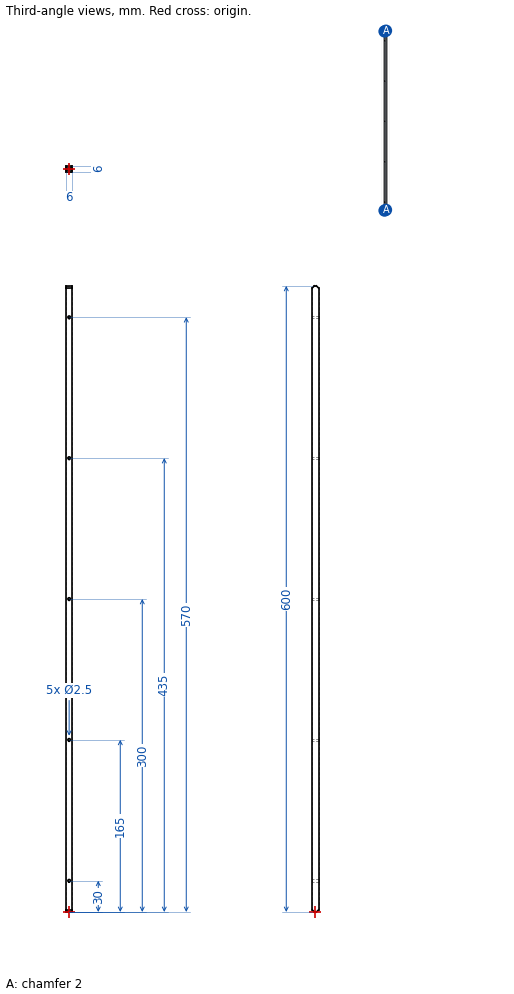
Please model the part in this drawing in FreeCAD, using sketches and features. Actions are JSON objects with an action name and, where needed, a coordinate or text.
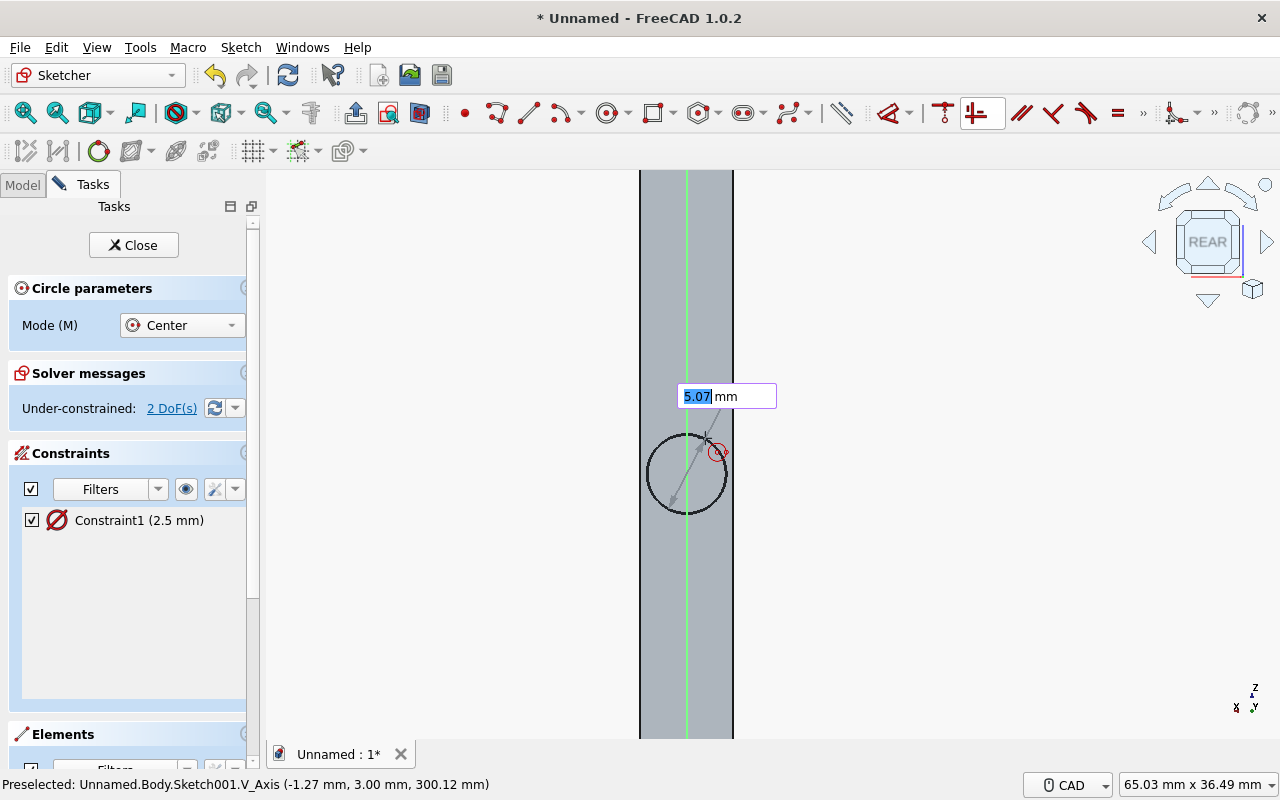
{"action": "type", "text": "2.5"}
{"action": "key", "text": "Return"}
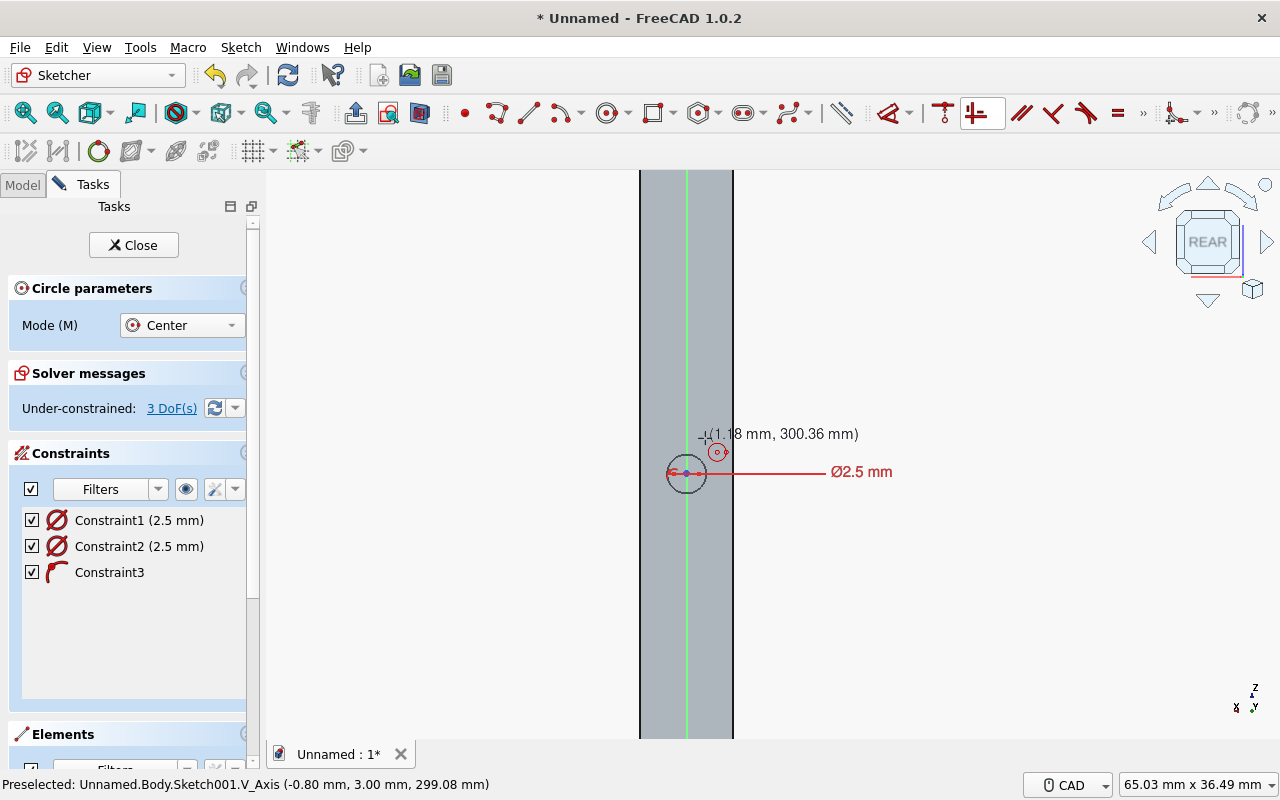
{"action": "scroll", "coordinate": [705, 443], "scroll_direction": "down", "scroll_amount": 15}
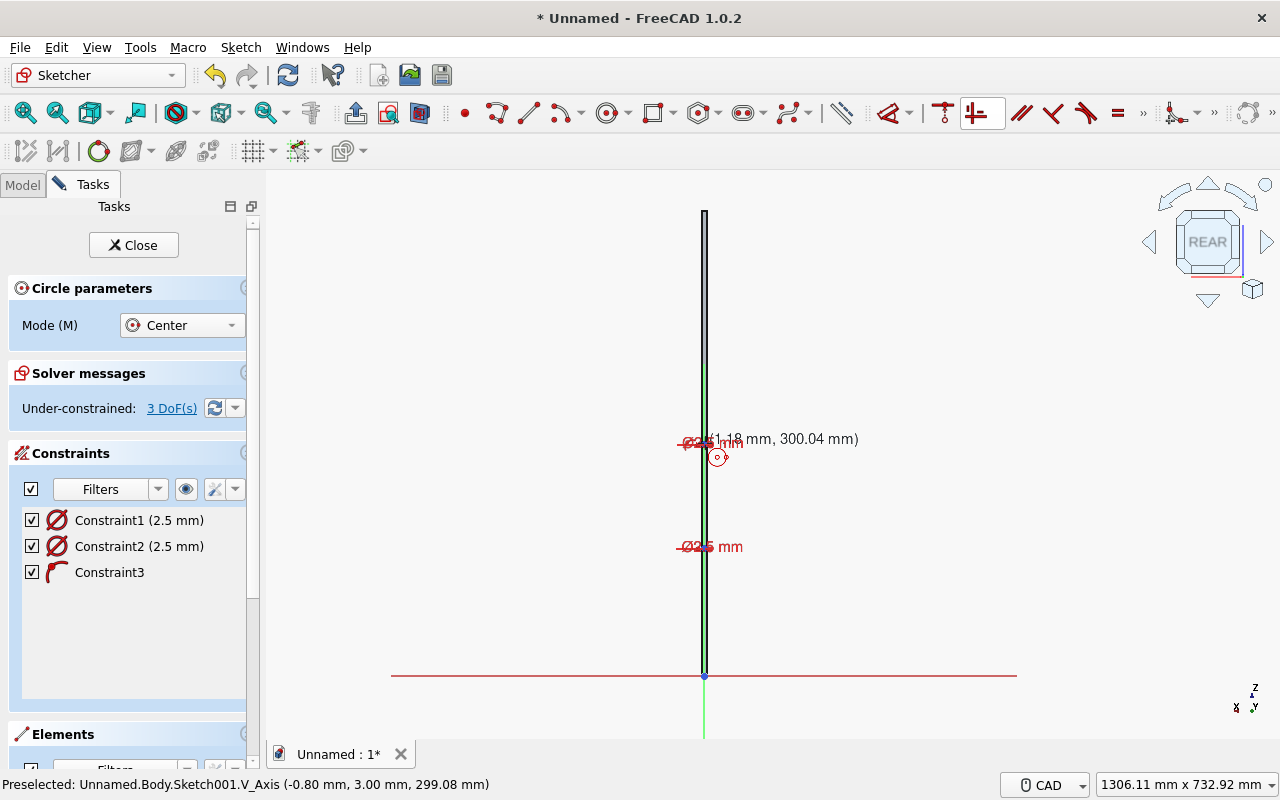
{"action": "scroll", "coordinate": [704, 339], "scroll_direction": "up", "scroll_amount": 16}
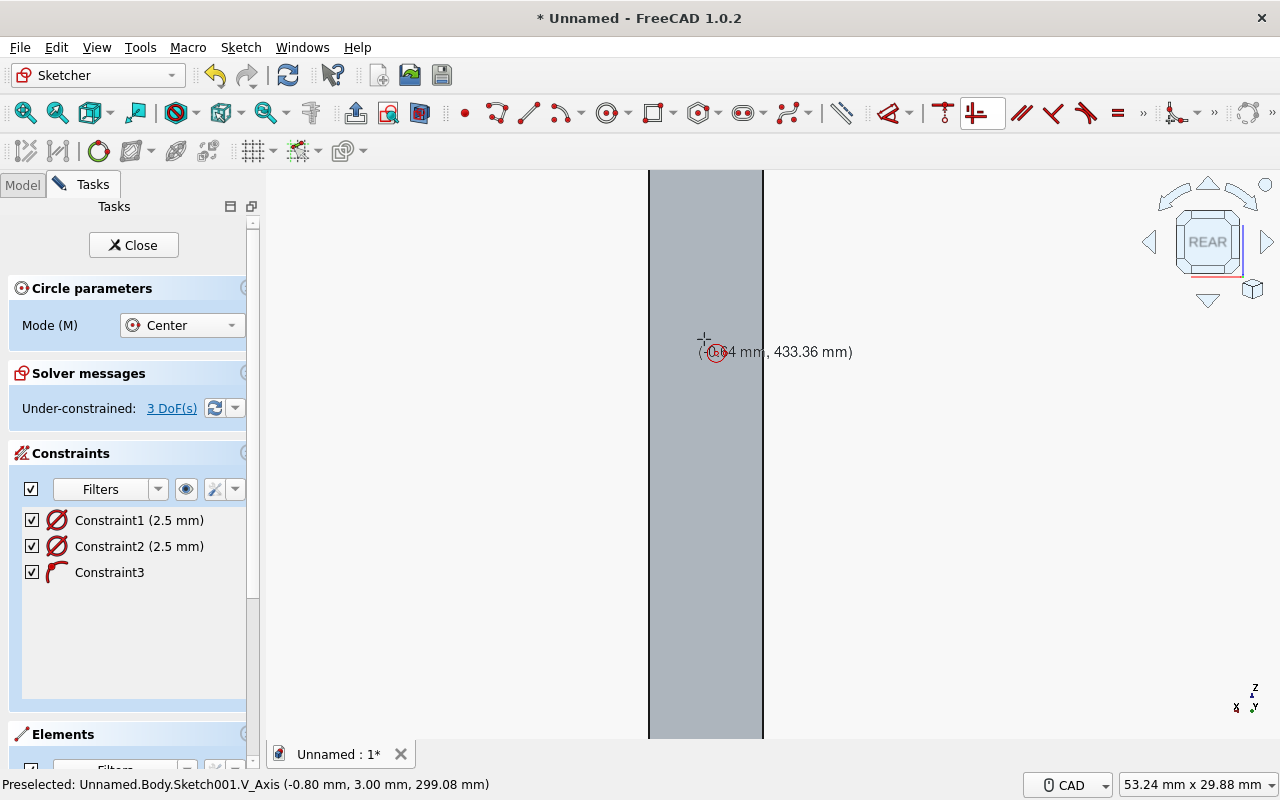
{"action": "scroll", "coordinate": [704, 339], "scroll_direction": "down", "scroll_amount": 16}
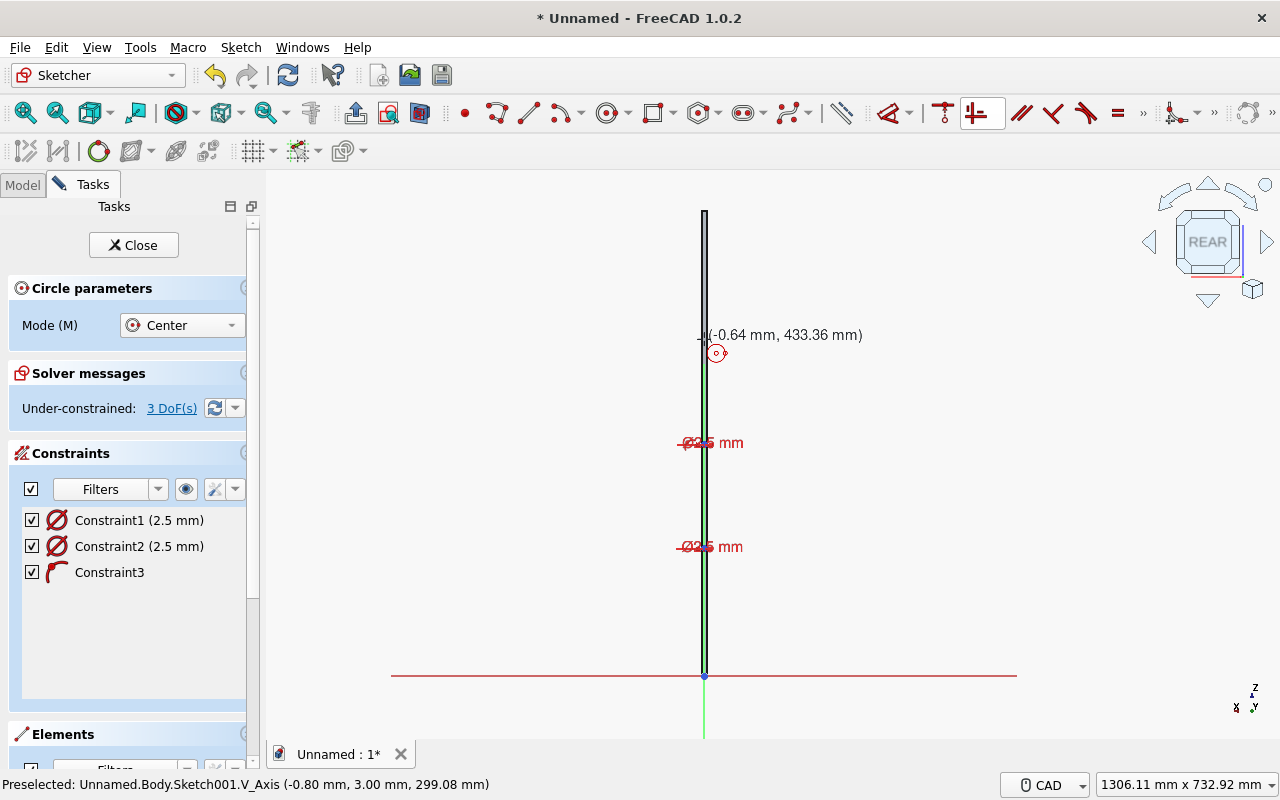
{"action": "left_click", "coordinate": [704, 339]}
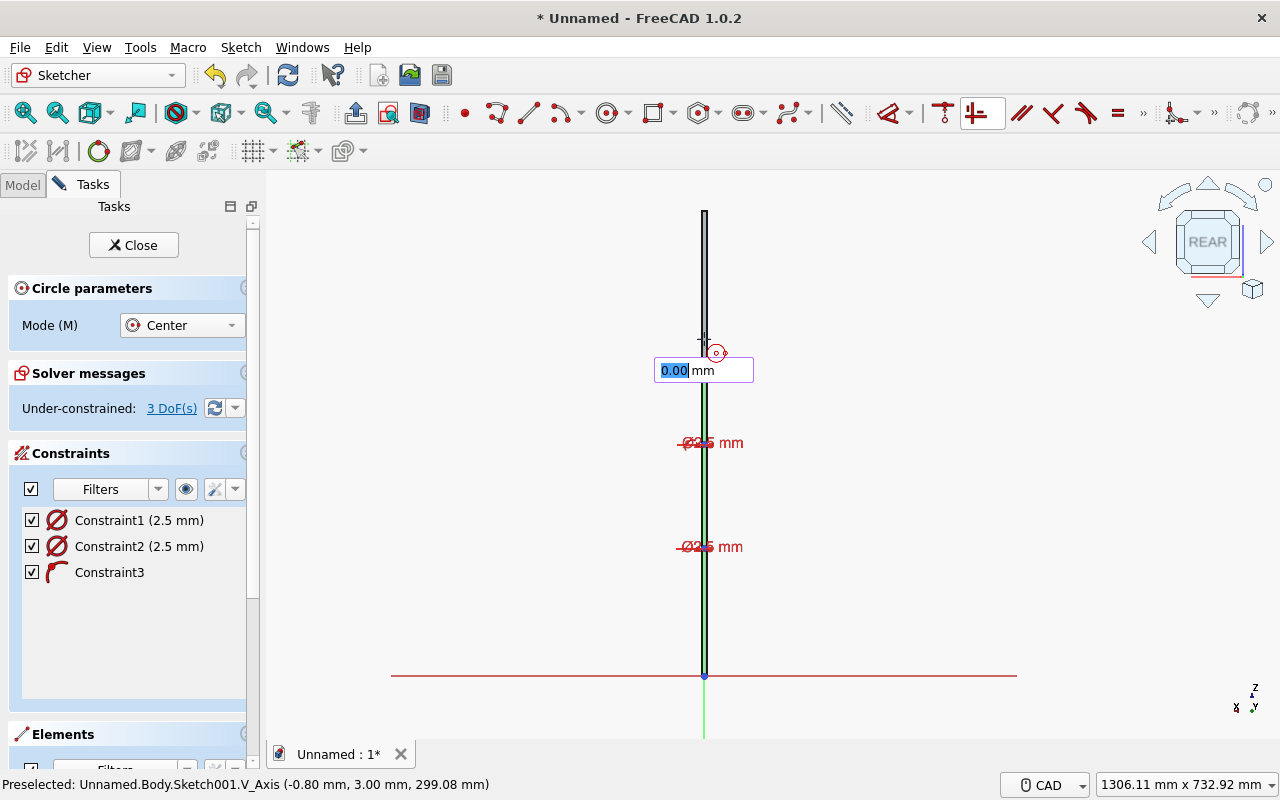
{"action": "scroll", "coordinate": [705, 338], "scroll_direction": "up", "scroll_amount": 15}
{"action": "mouse_move", "coordinate": [705, 340]}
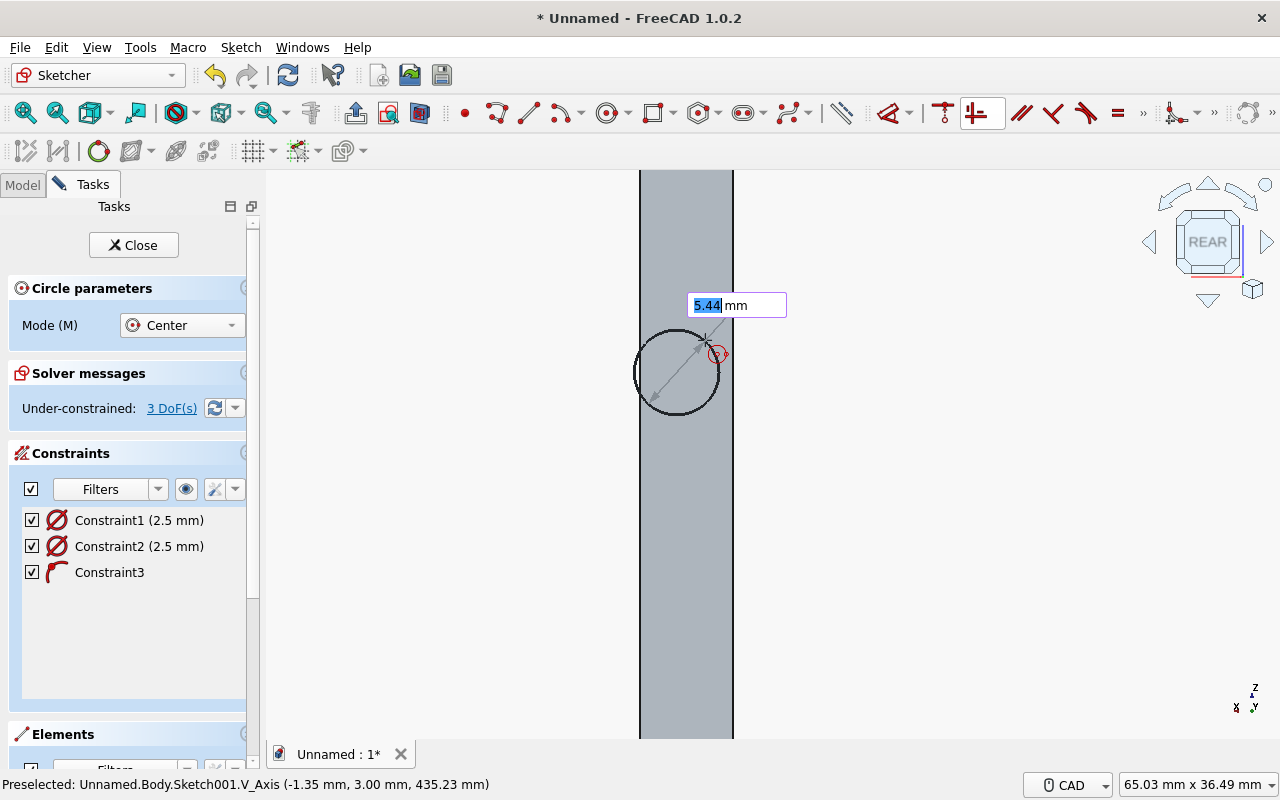
{"action": "type", "text": "2.5"}
{"action": "key", "text": "Return"}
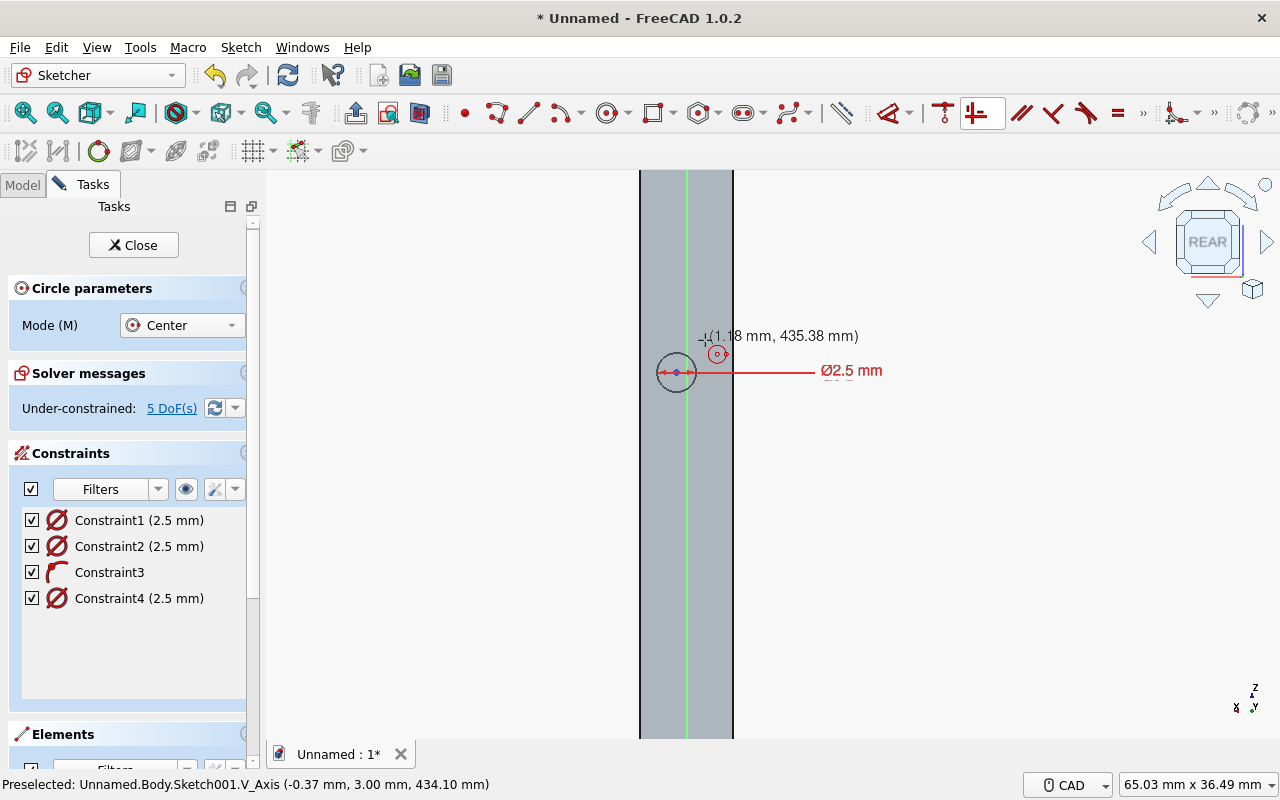
{"action": "scroll", "coordinate": [705, 338], "scroll_direction": "down", "scroll_amount": 15}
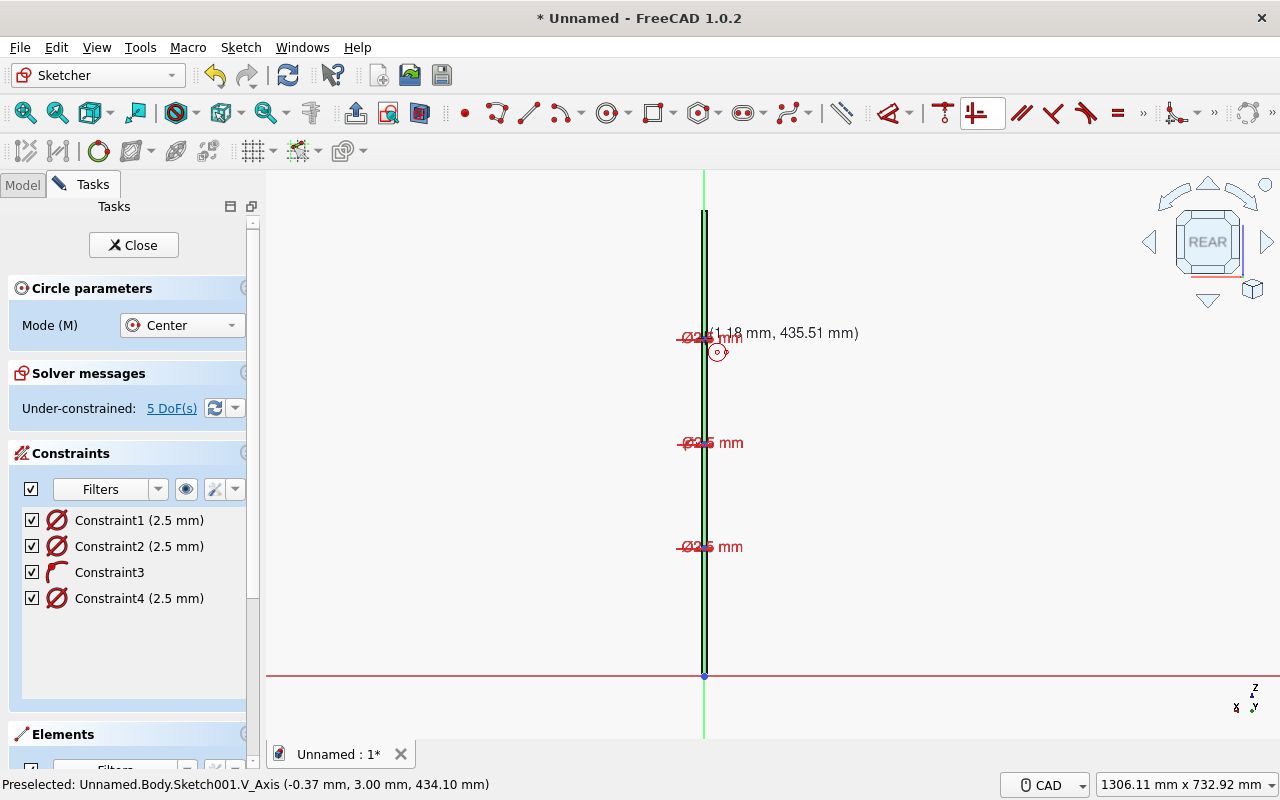
{"action": "scroll", "coordinate": [704, 234], "scroll_direction": "up", "scroll_amount": 16}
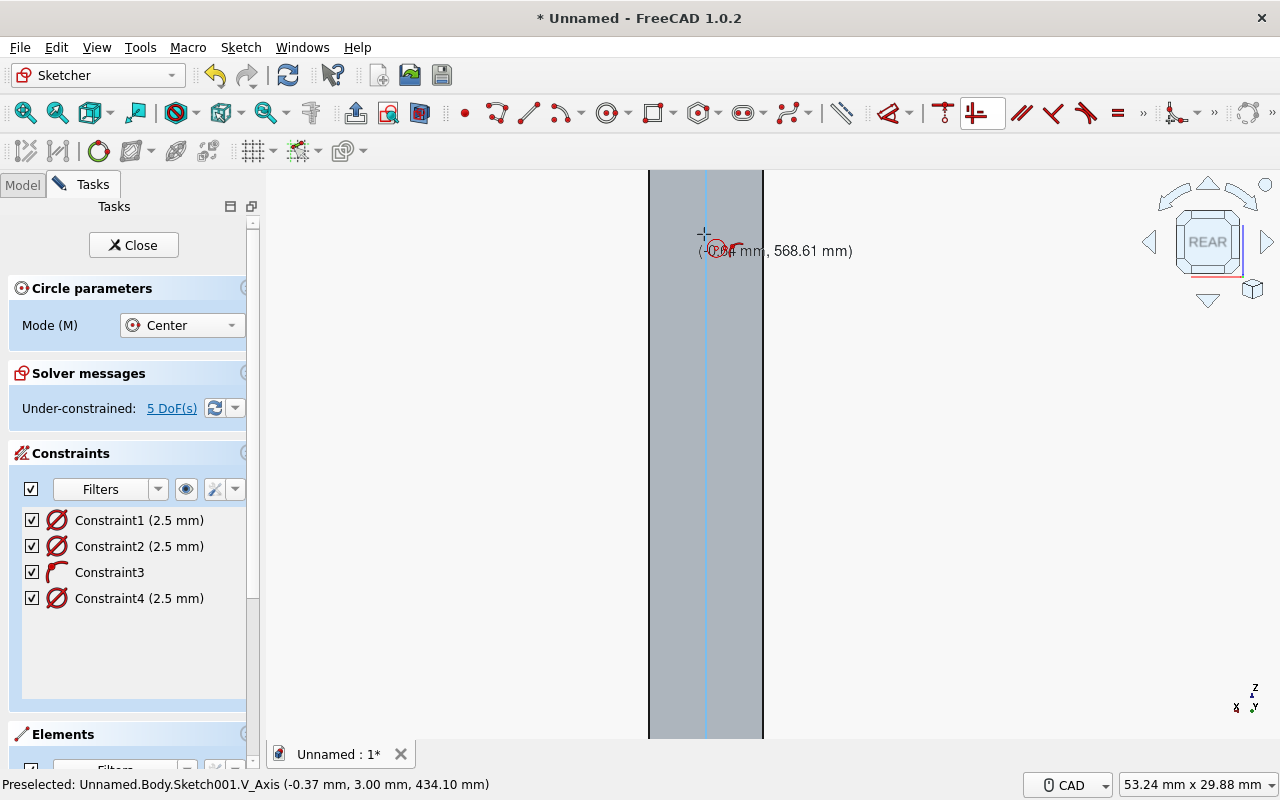
{"action": "scroll", "coordinate": [704, 234], "scroll_direction": "down", "scroll_amount": 16}